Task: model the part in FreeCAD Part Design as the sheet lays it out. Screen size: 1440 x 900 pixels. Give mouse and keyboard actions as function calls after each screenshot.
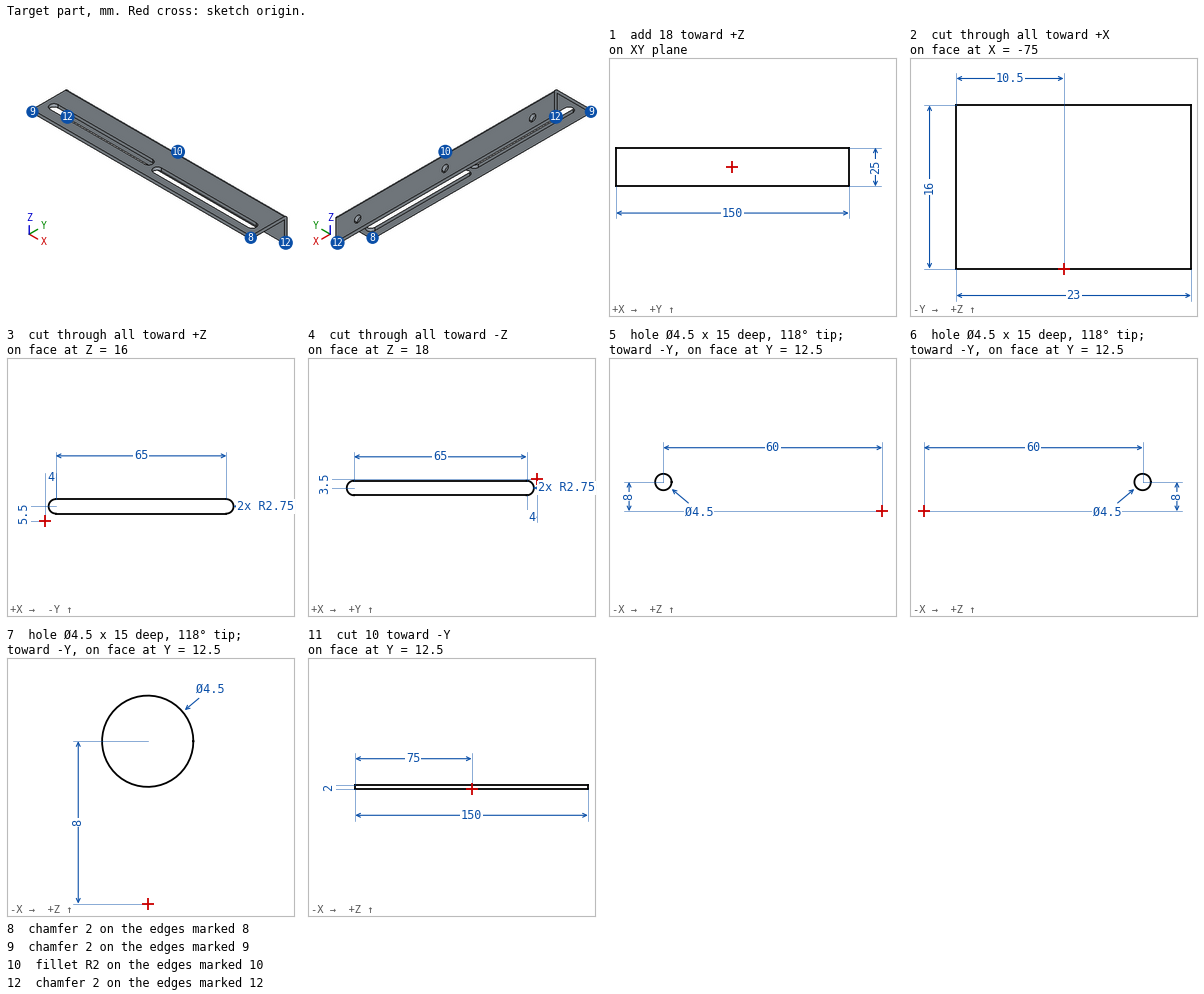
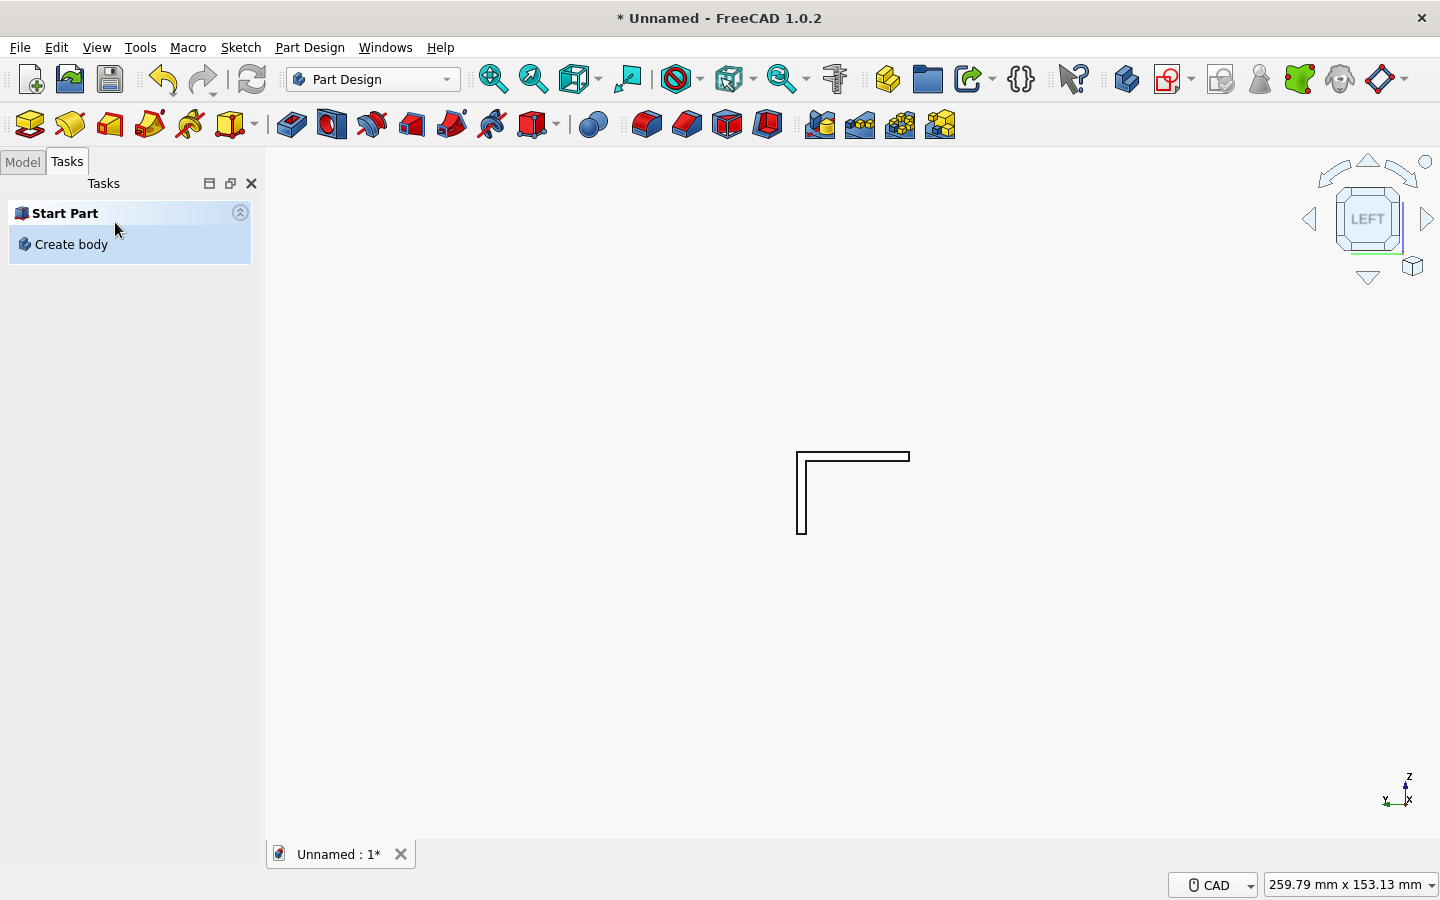
click(494, 80)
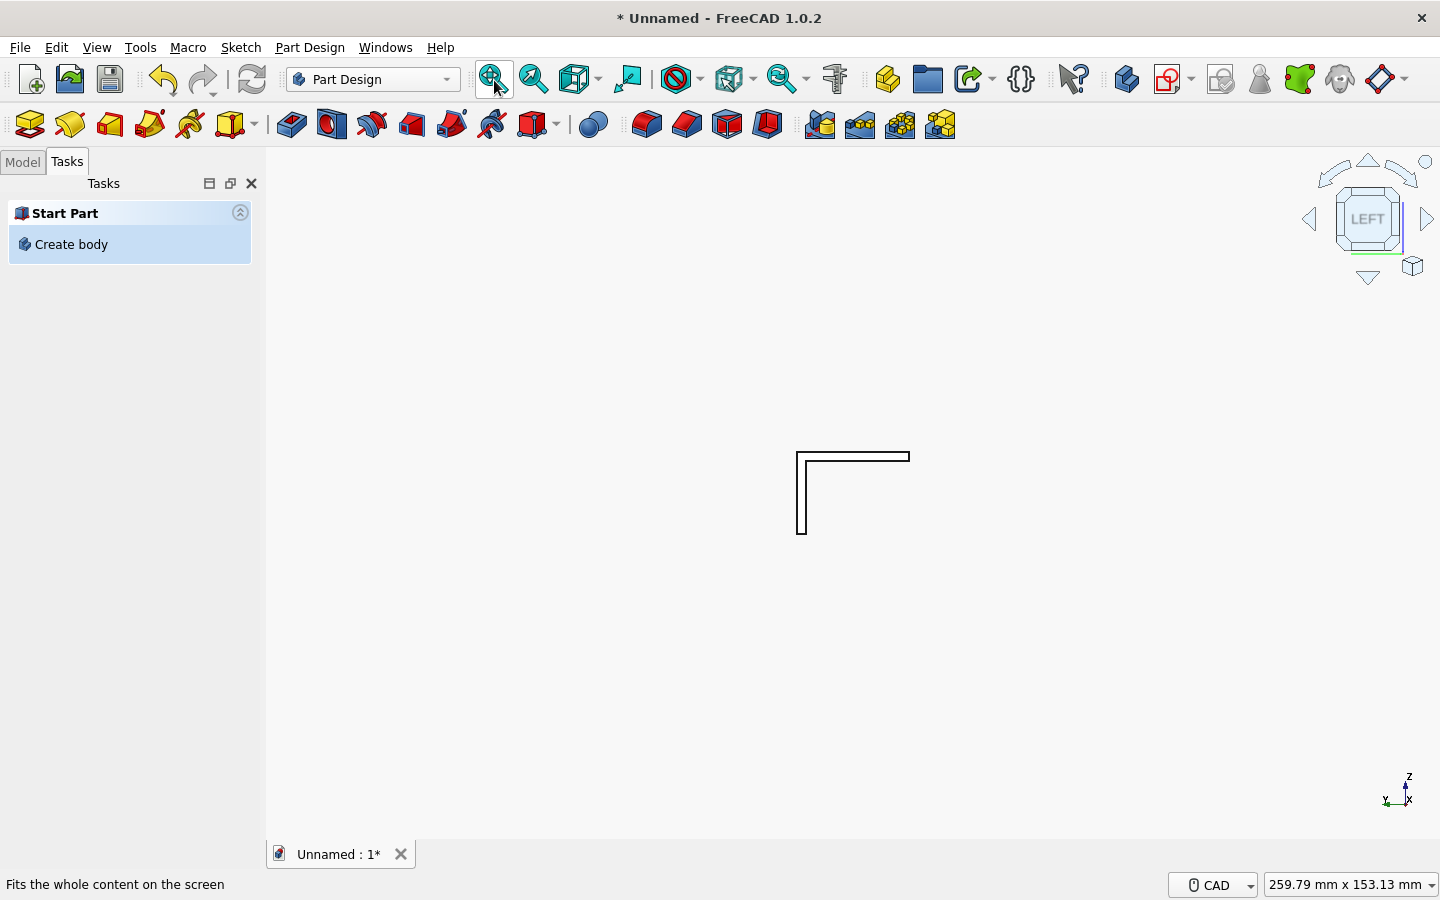
key(5)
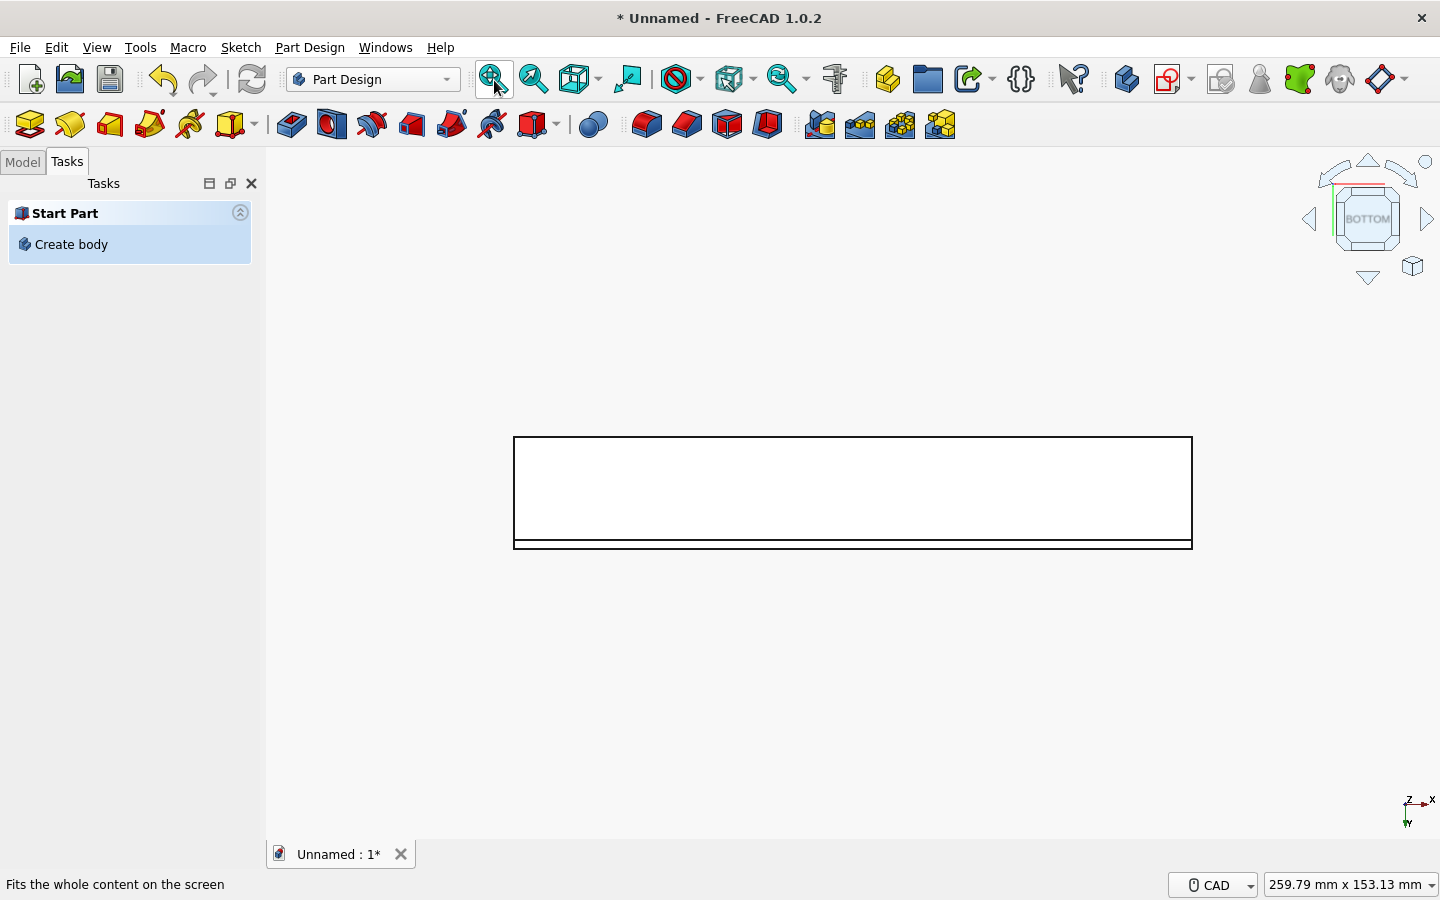
click(1047, 487)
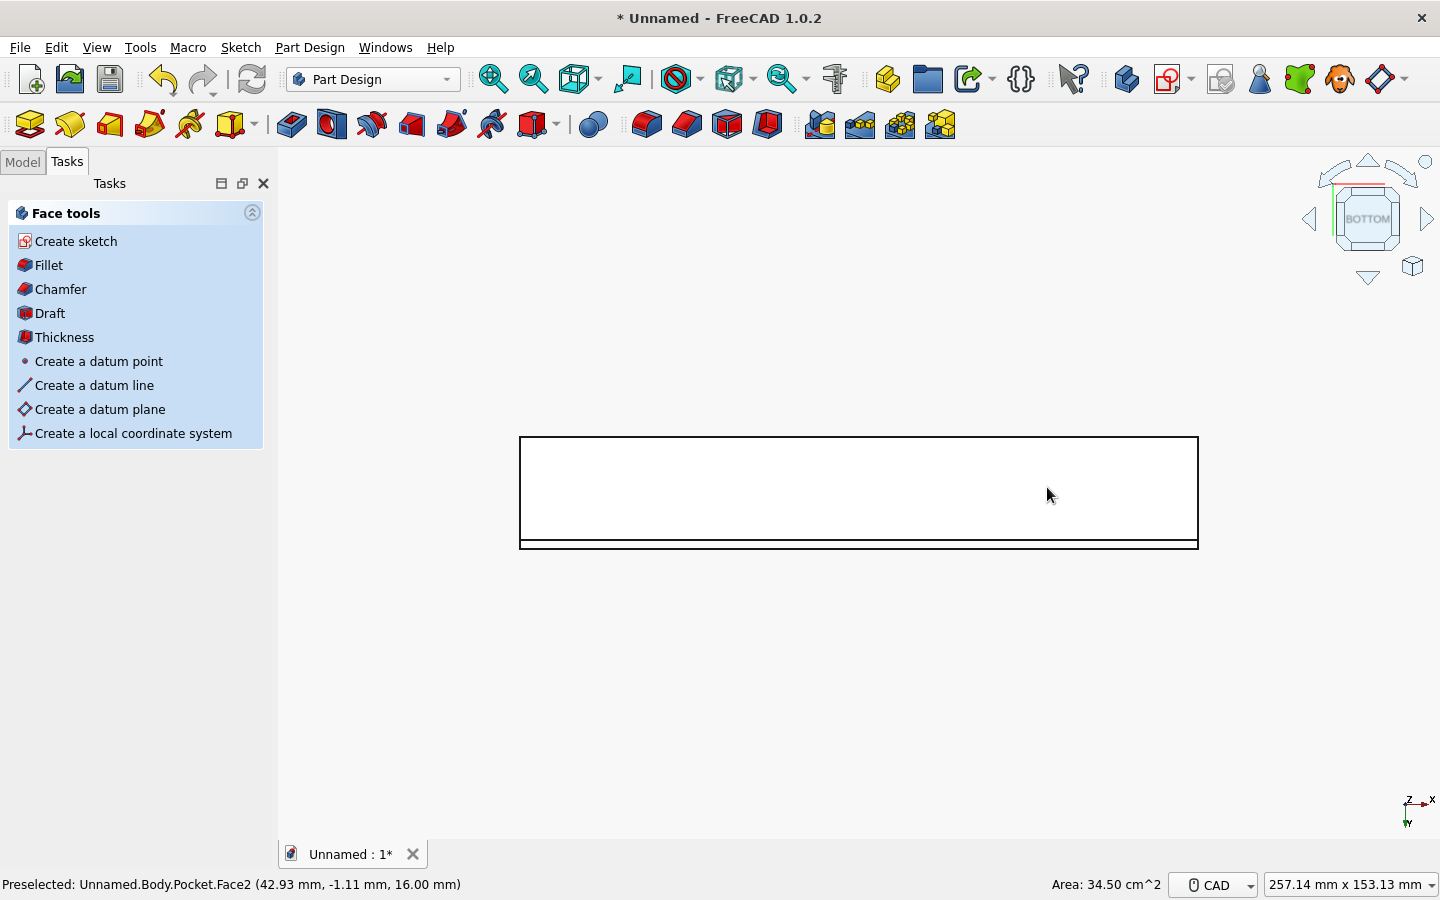
click(1168, 80)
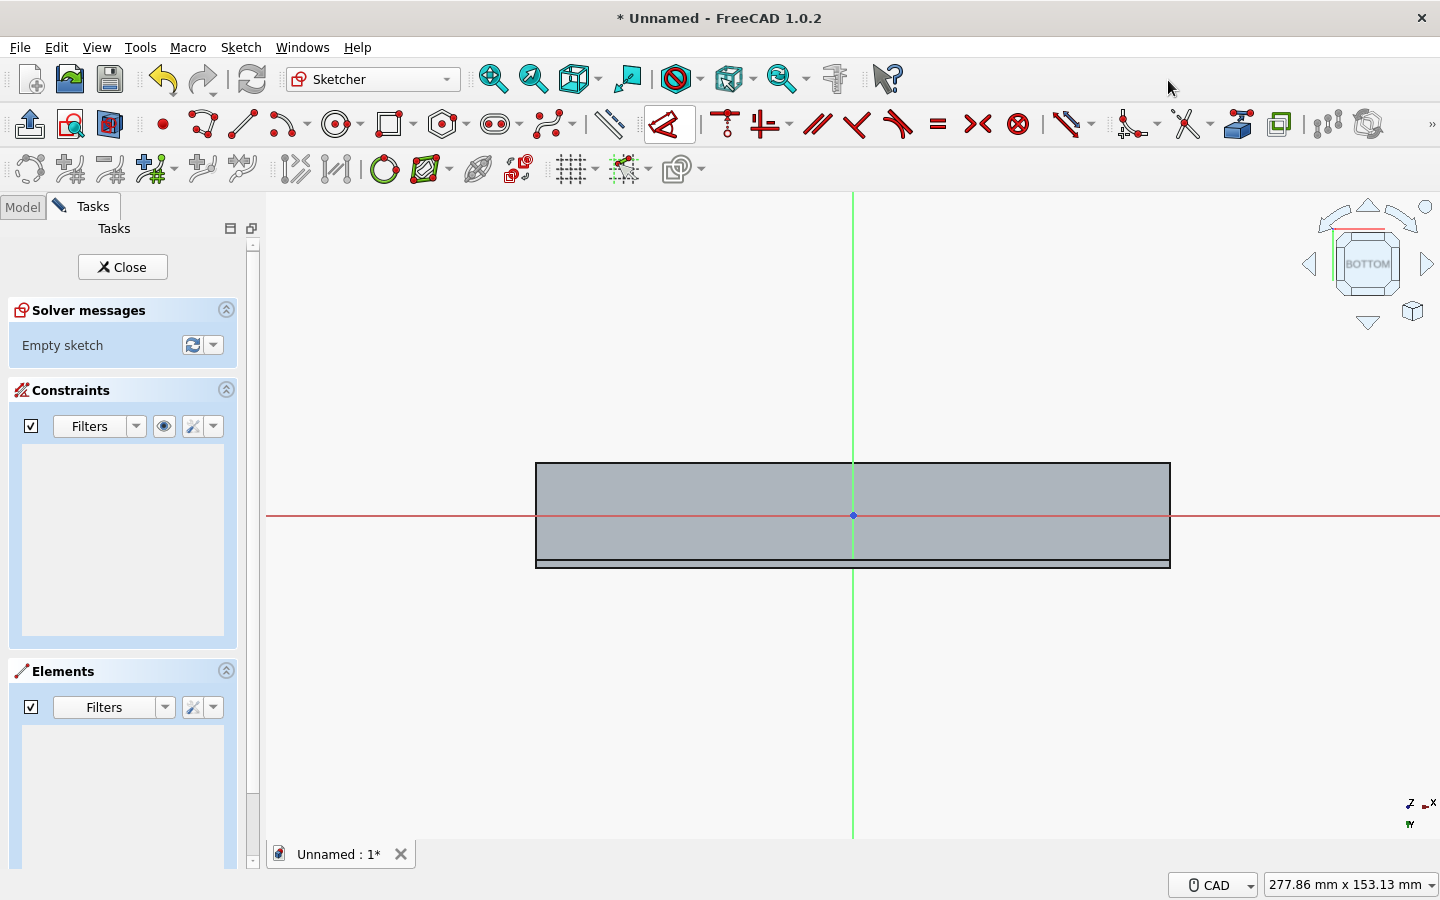
scroll(1184, 484, up, 4)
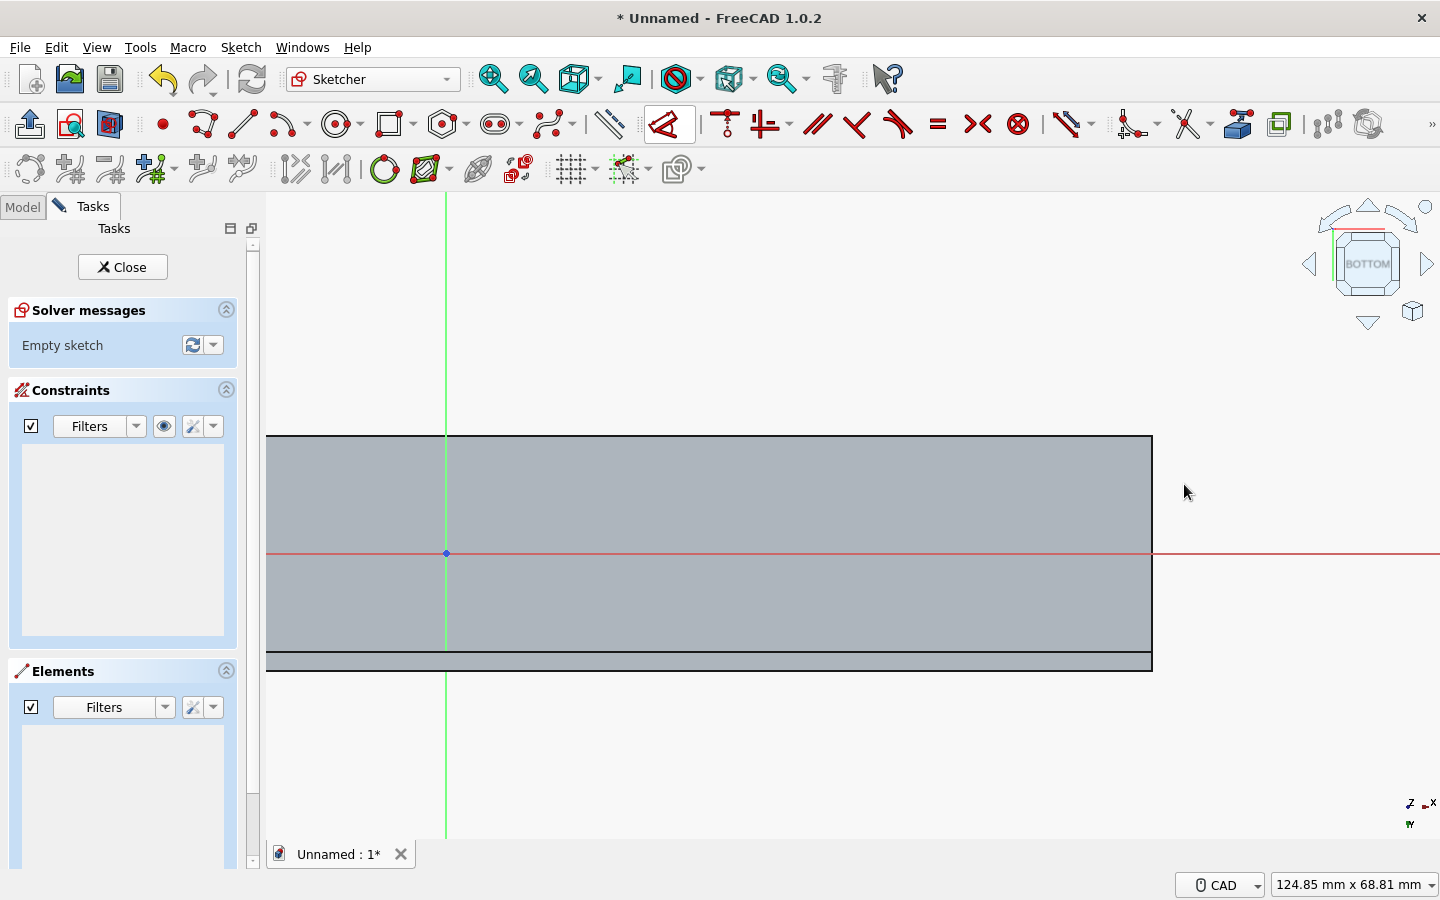
click(496, 124)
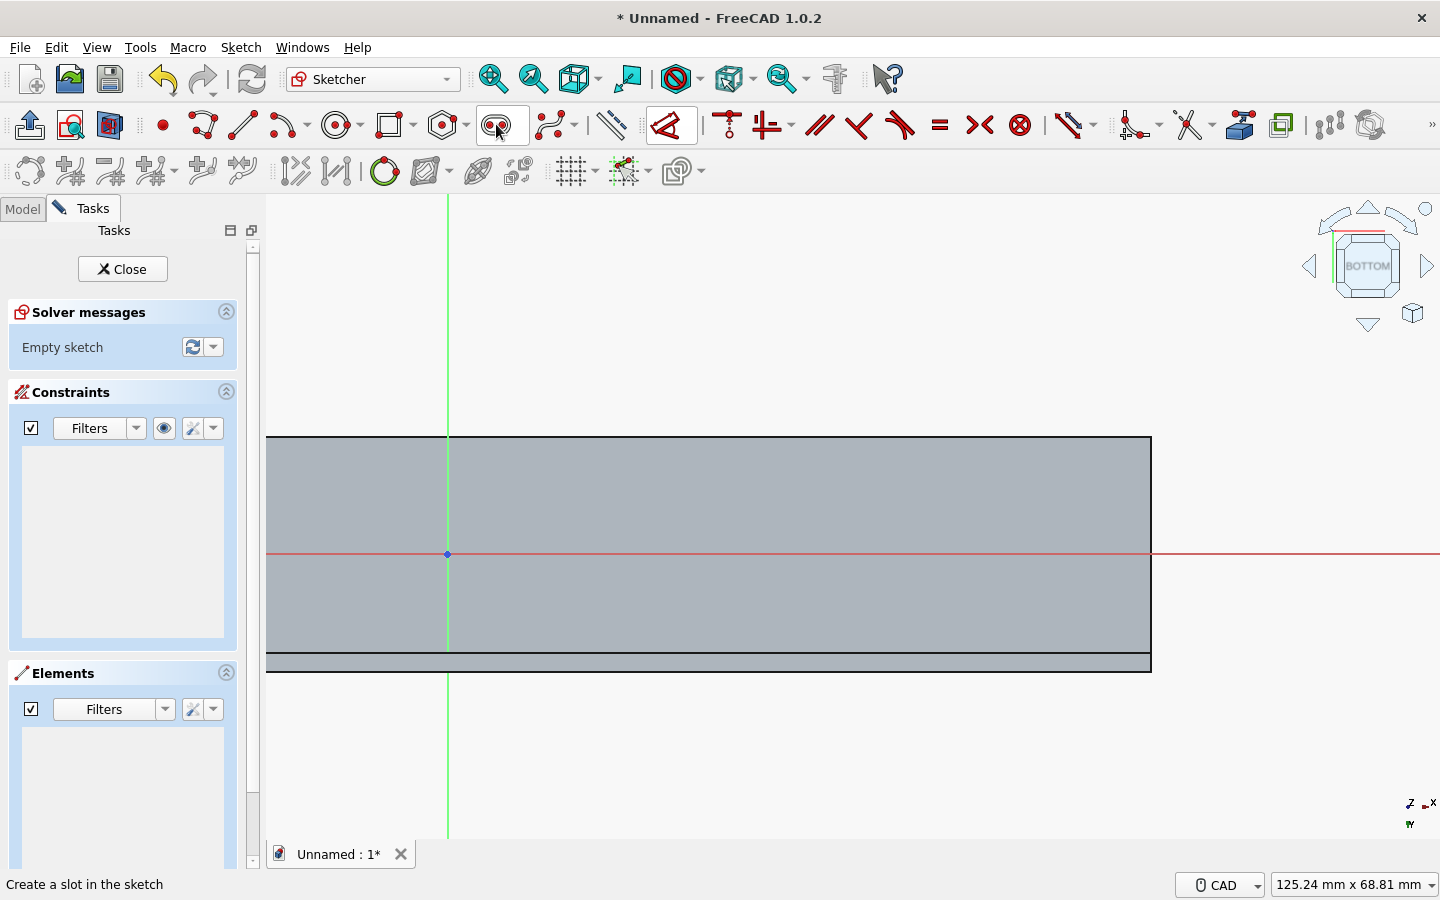
click(485, 503)